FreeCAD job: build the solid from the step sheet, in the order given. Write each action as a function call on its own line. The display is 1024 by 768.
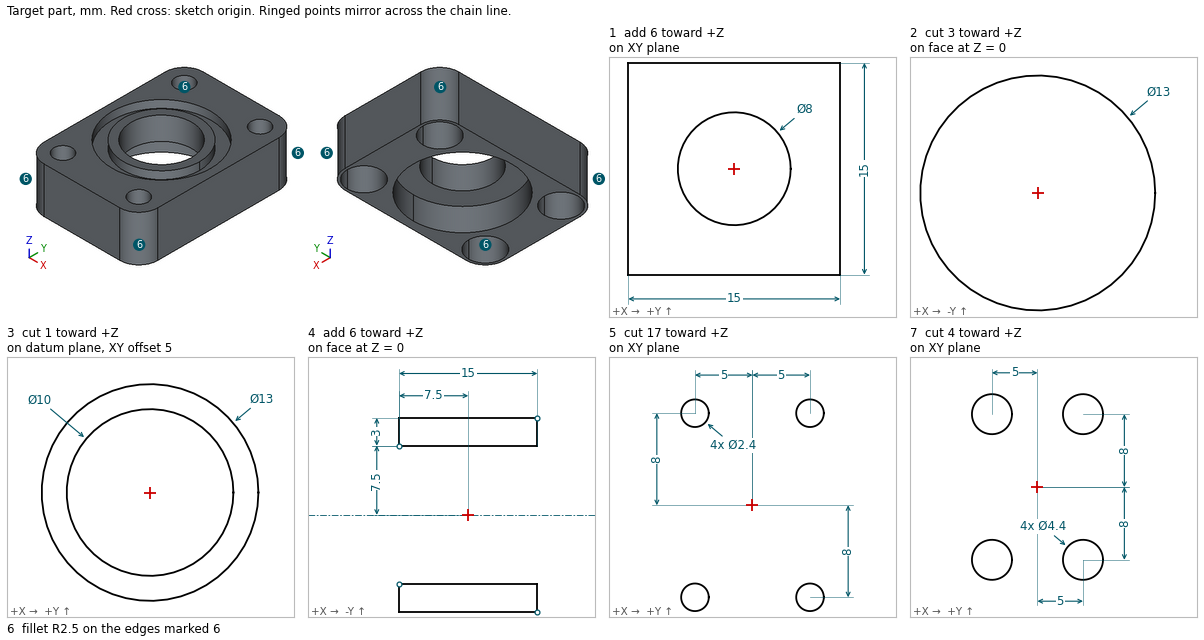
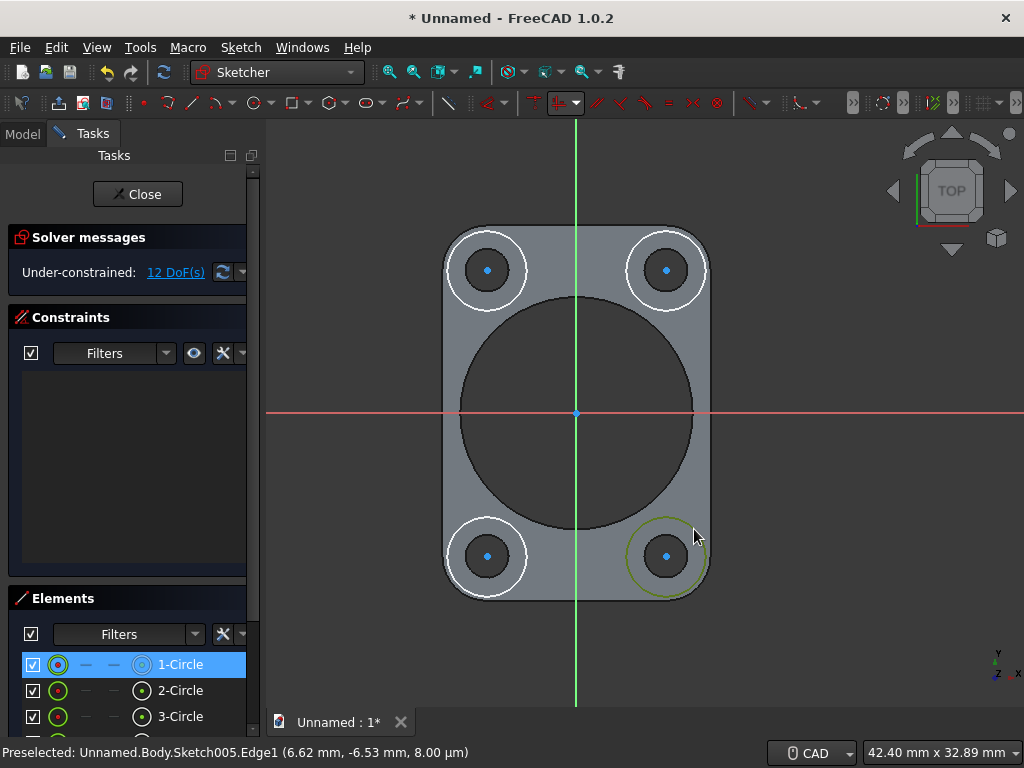
click(694, 243)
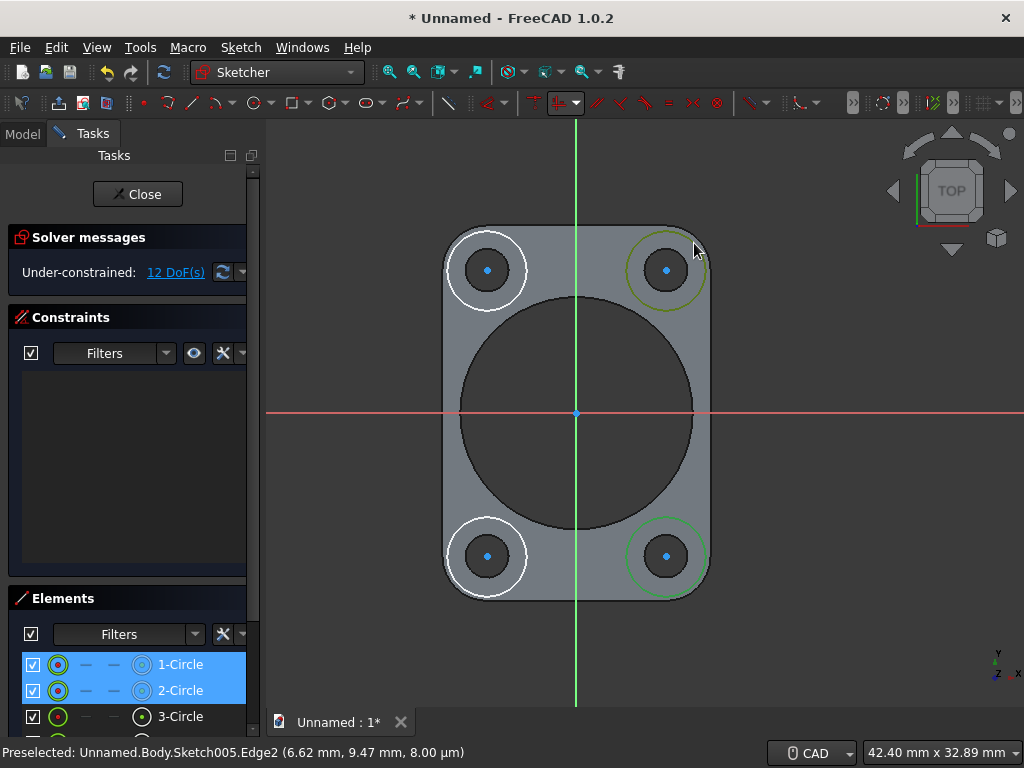
click(515, 243)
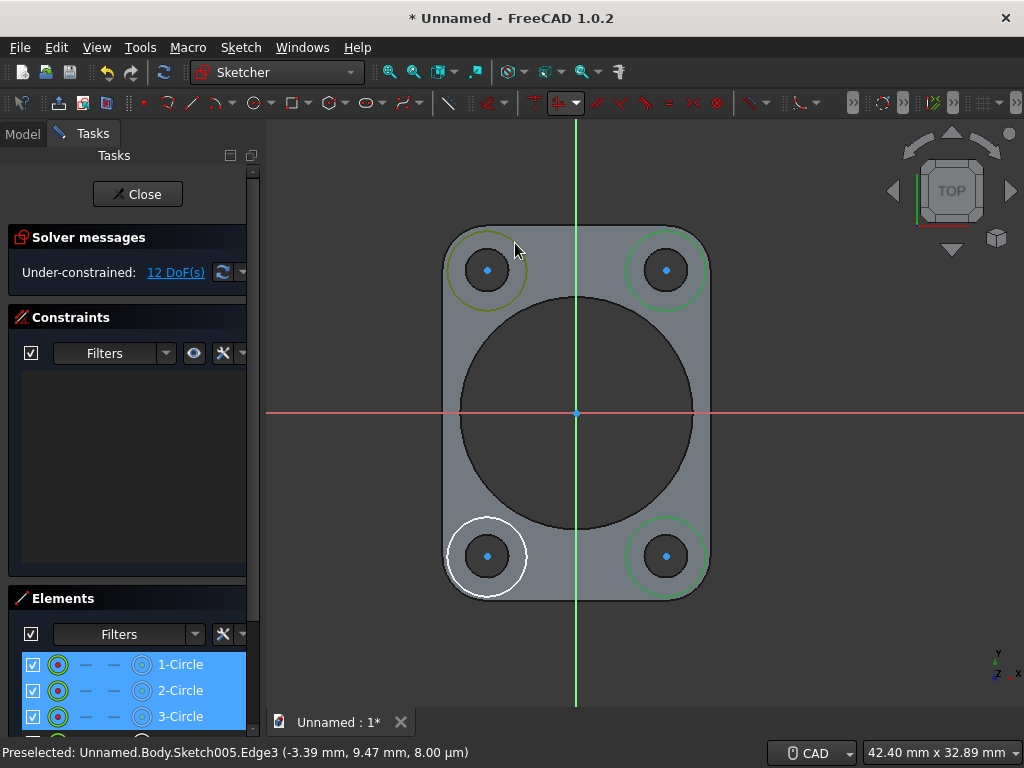
click(515, 529)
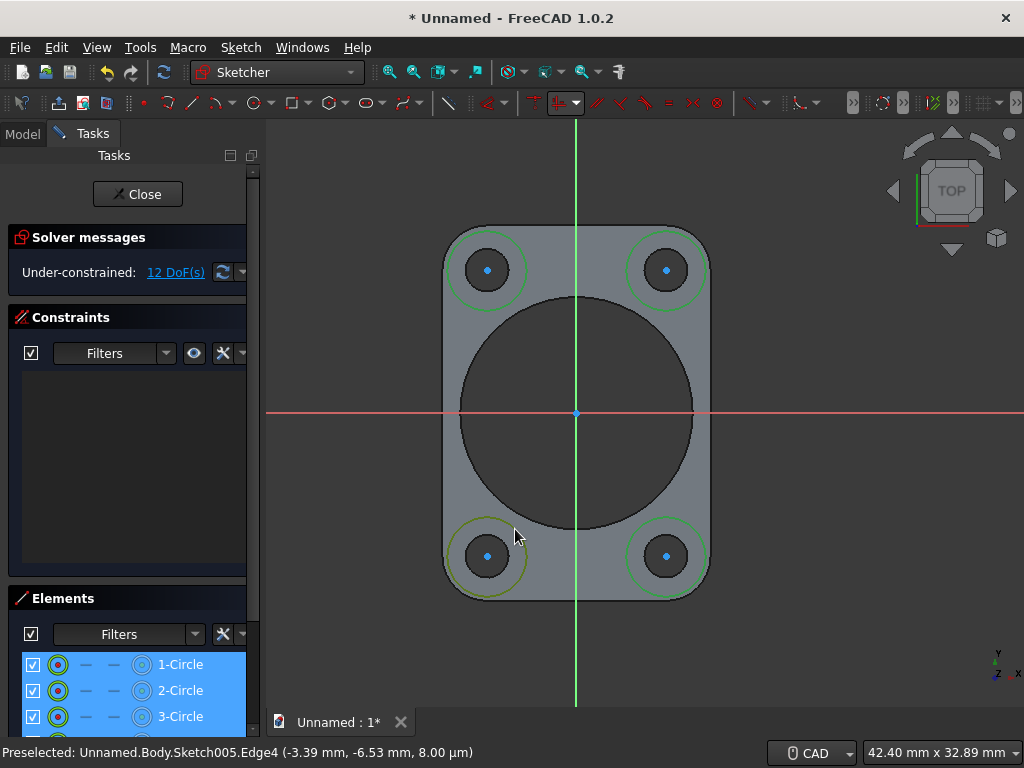
click(670, 104)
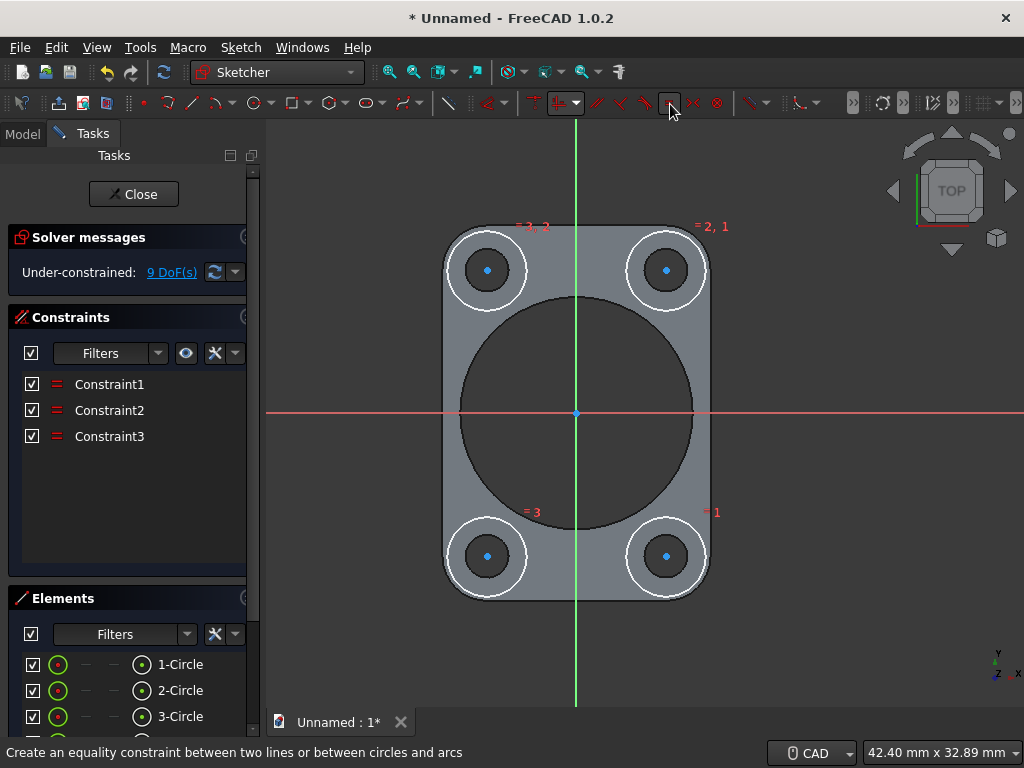
click(666, 557)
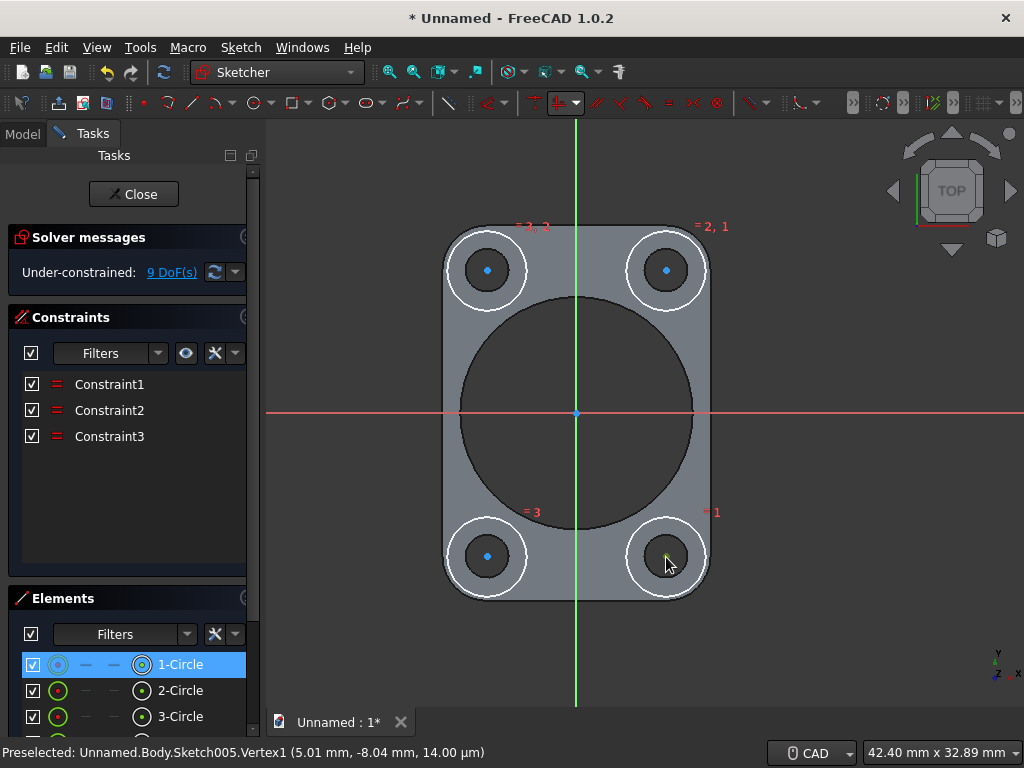
click(666, 271)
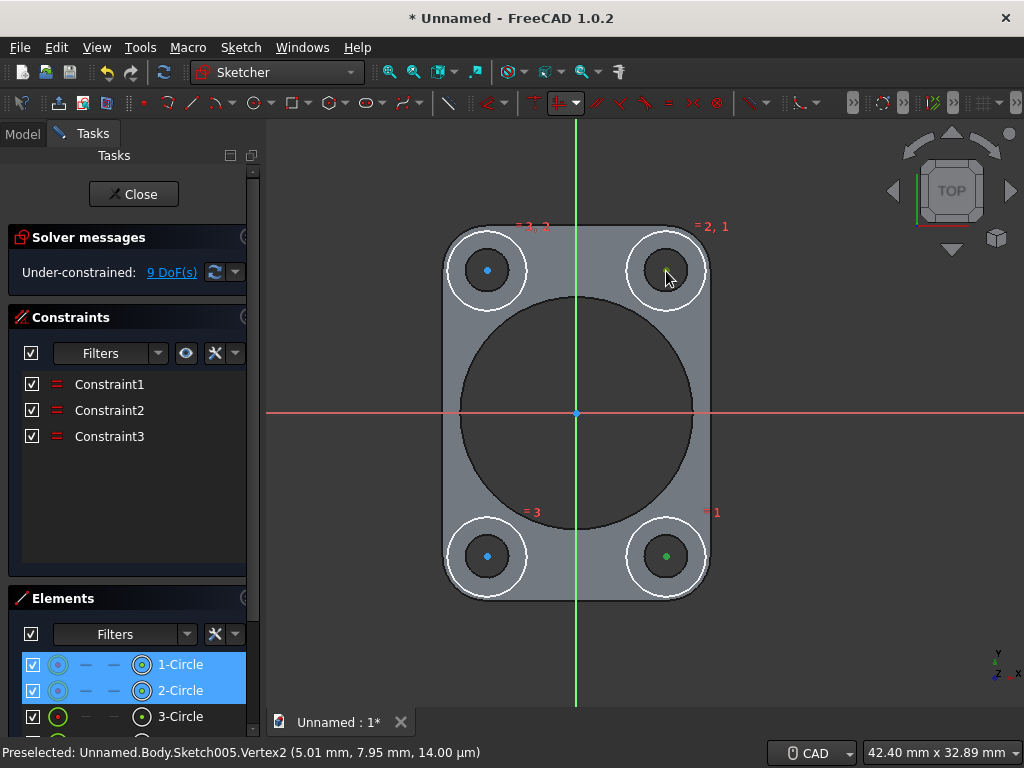
key(v)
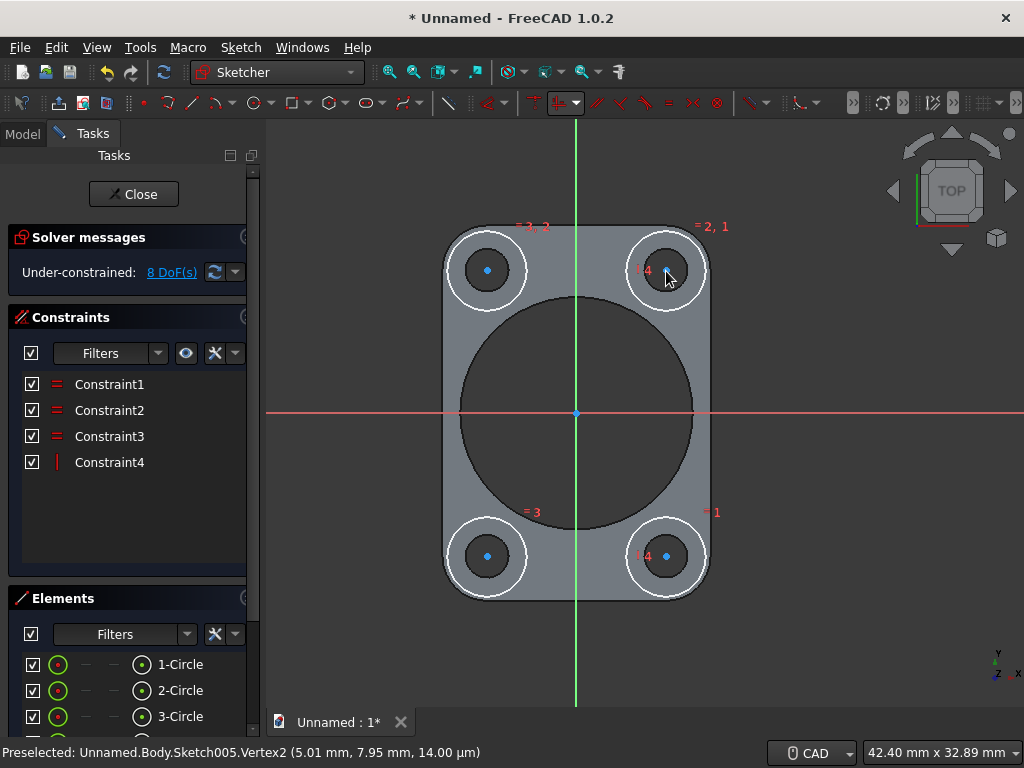
click(666, 271)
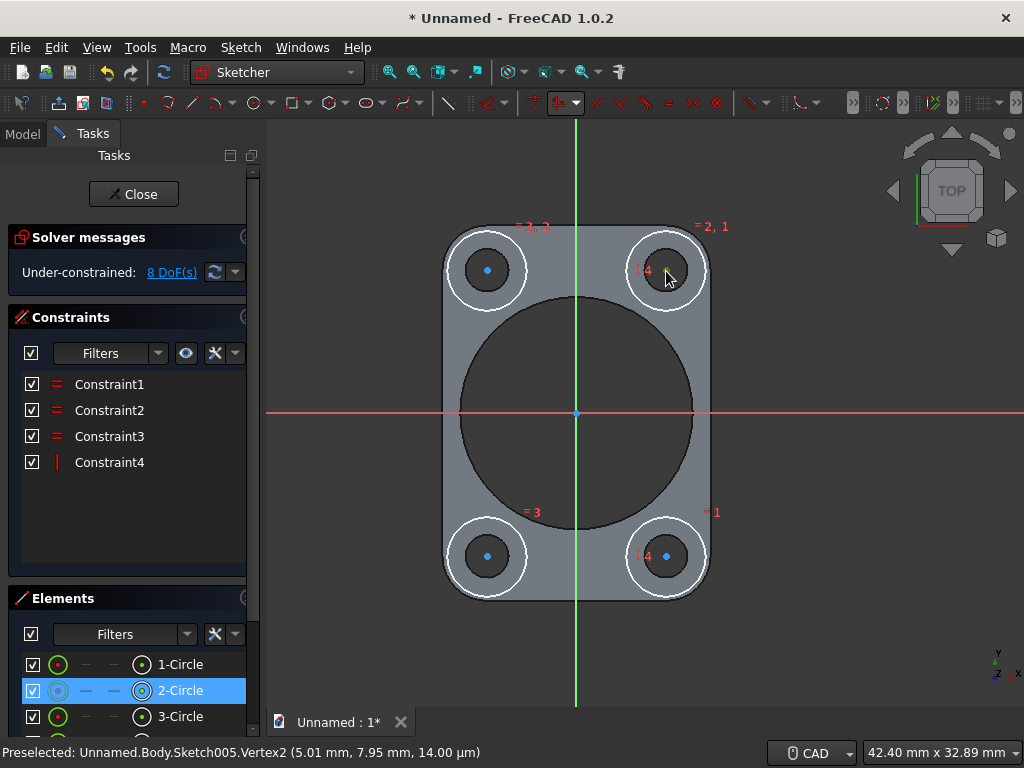
click(487, 271)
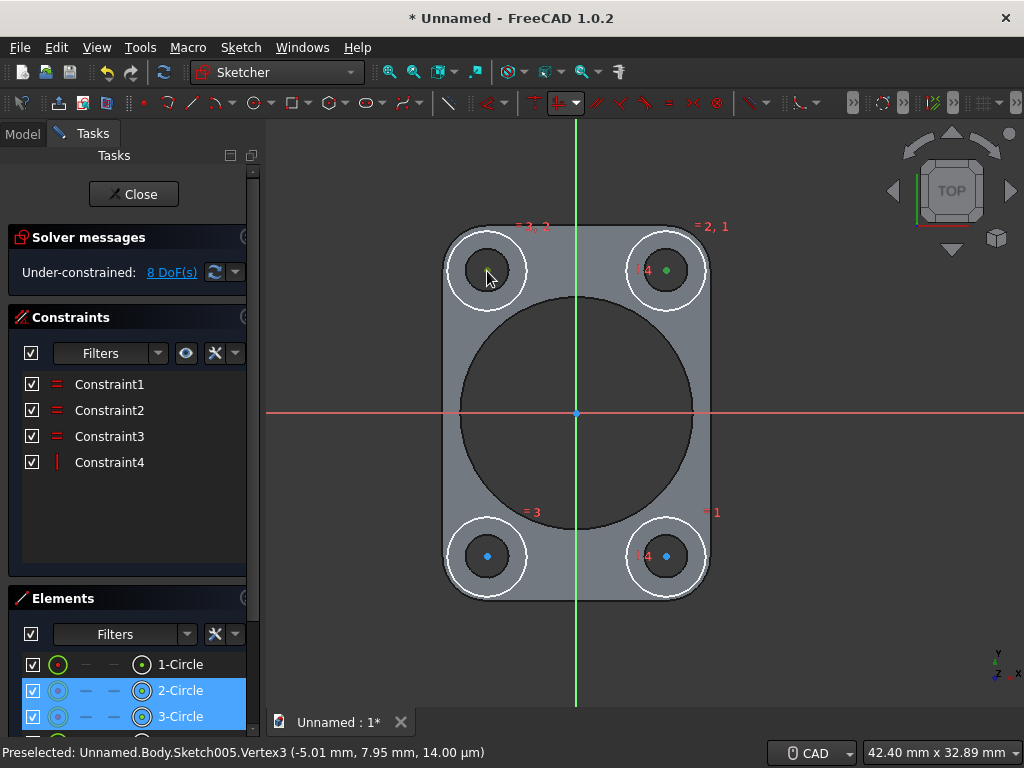
key(h)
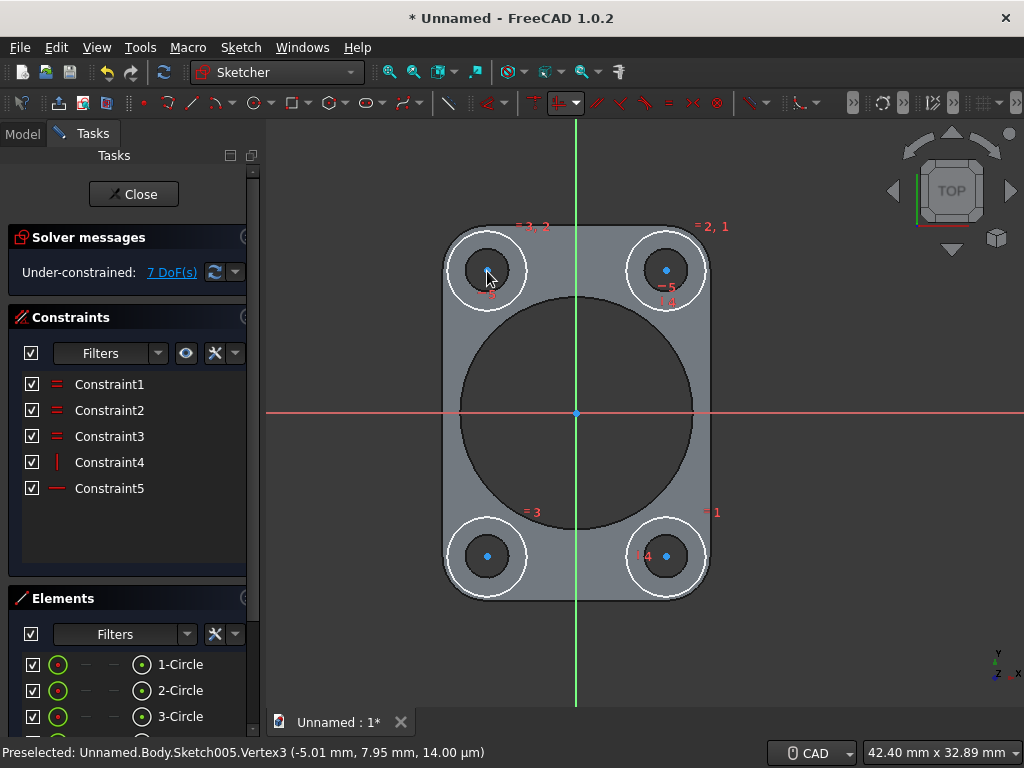
click(487, 271)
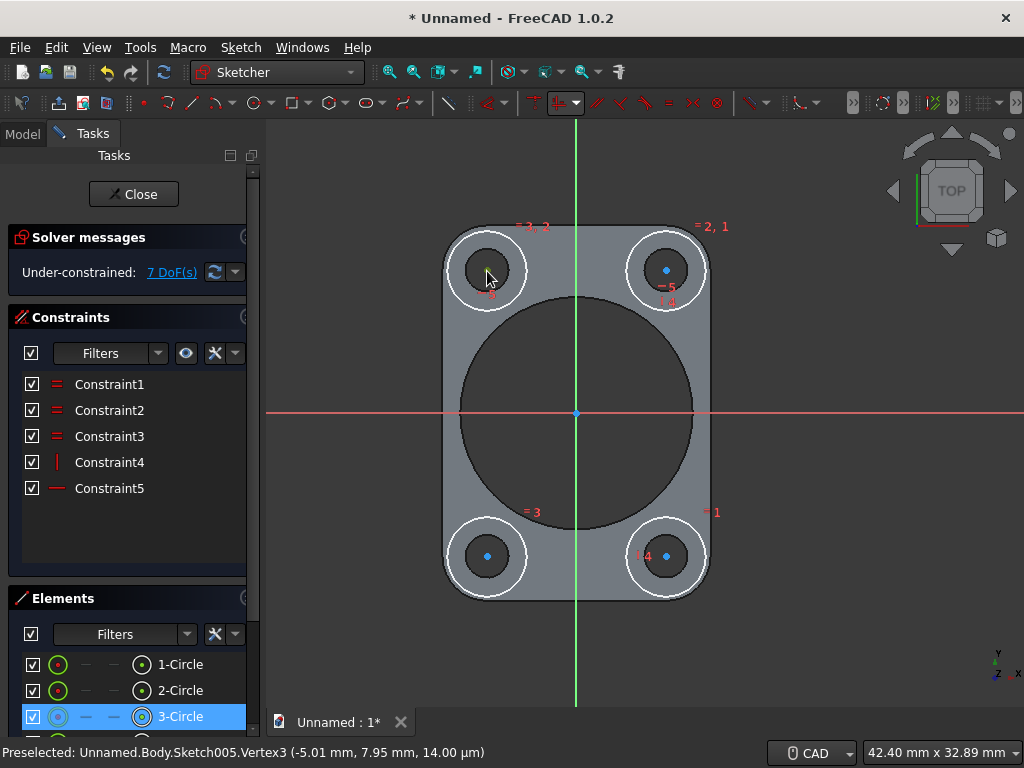
click(487, 557)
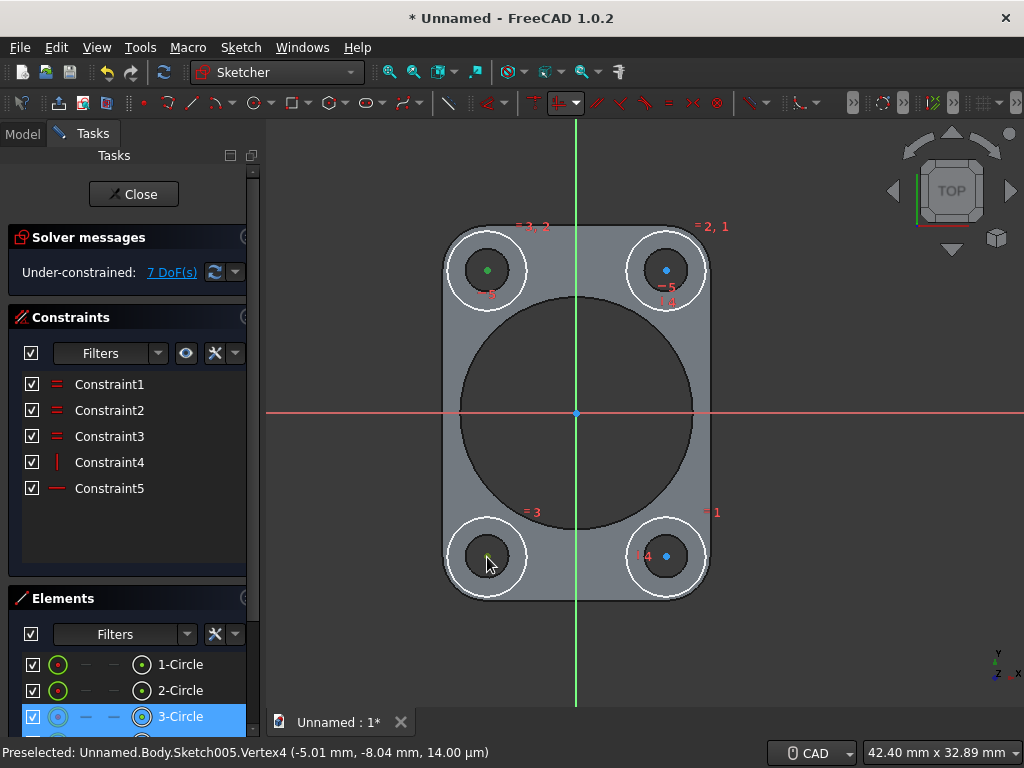
click(578, 104)